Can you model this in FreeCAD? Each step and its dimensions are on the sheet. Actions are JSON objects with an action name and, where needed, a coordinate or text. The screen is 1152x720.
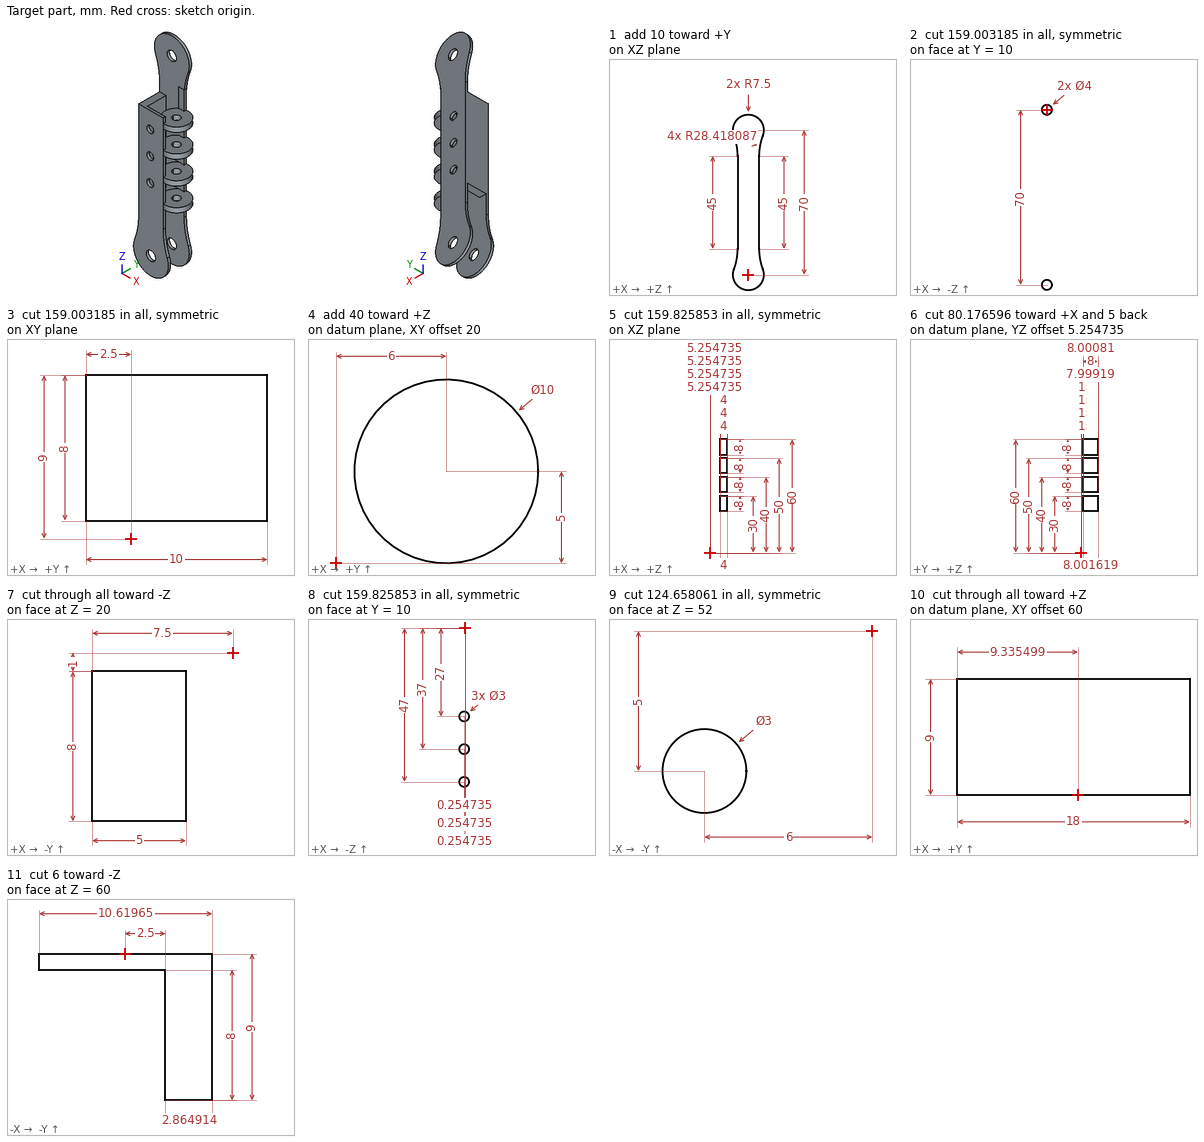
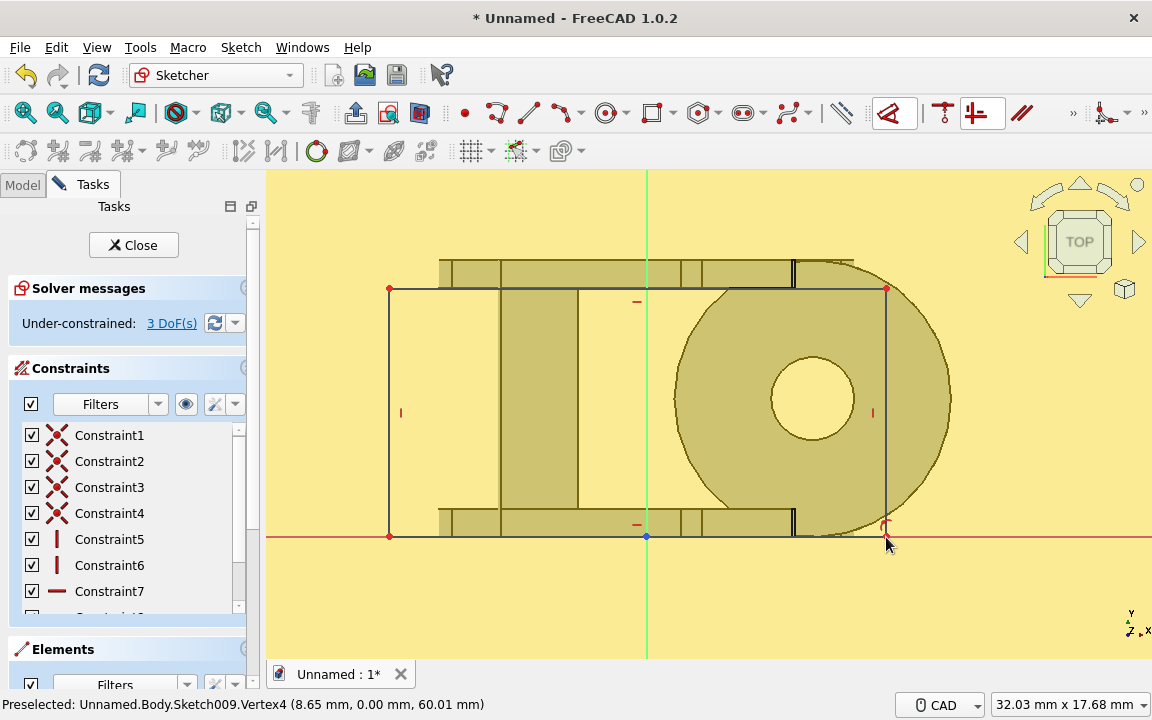
{"action": "left_click", "coordinate": [389, 363]}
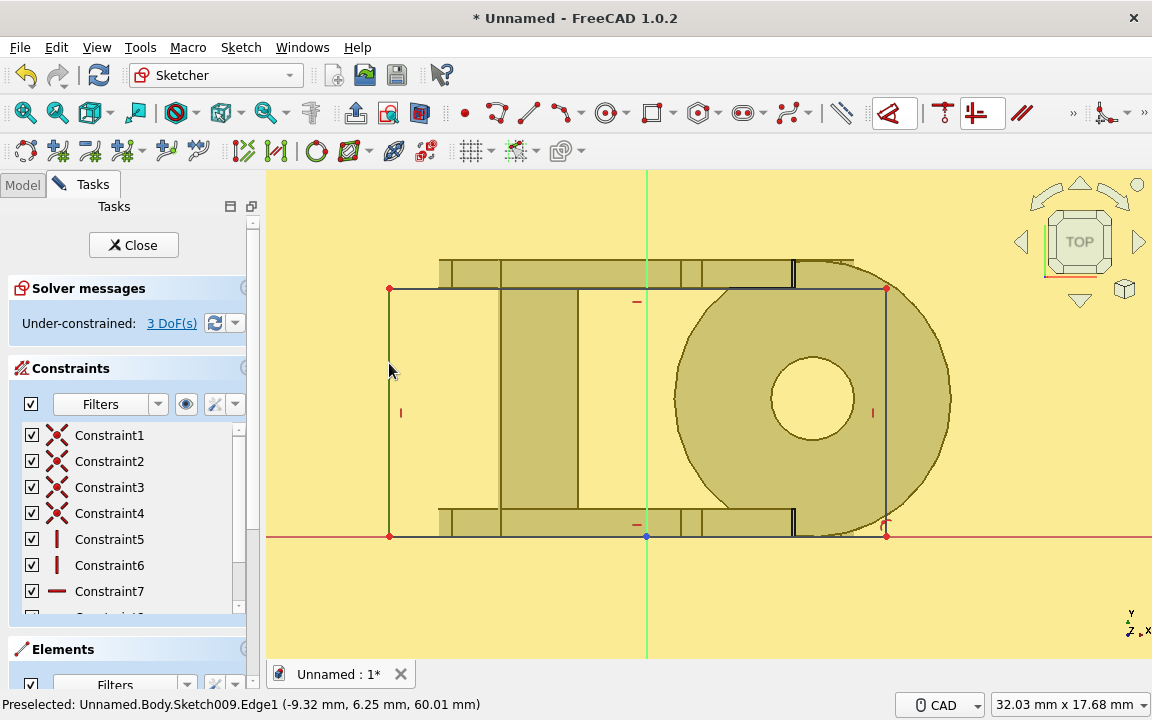
{"action": "key", "text": "i"}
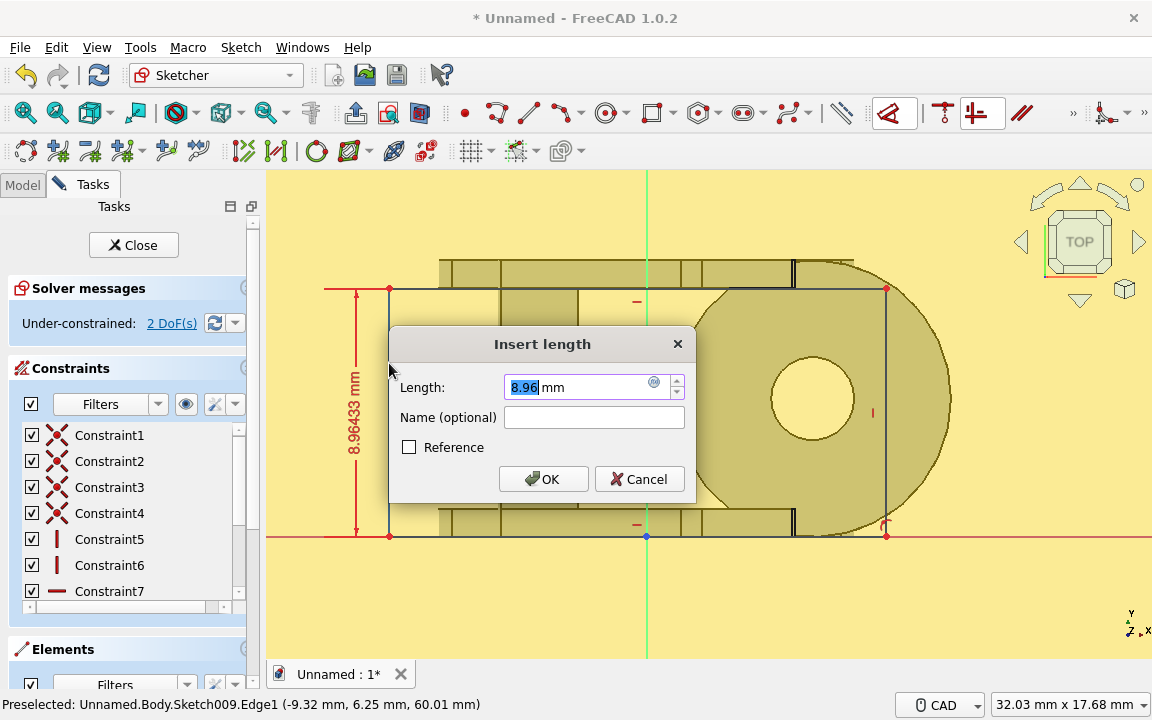
{"action": "type", "text": "9"}
{"action": "key", "text": "Return"}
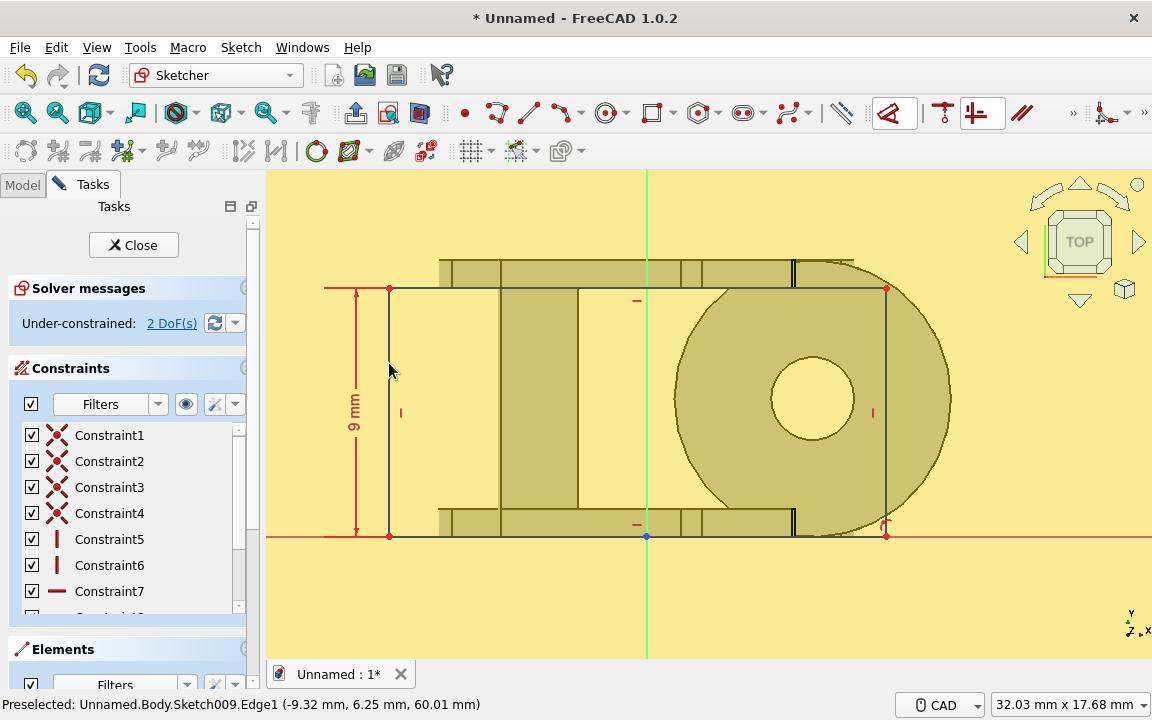
{"action": "left_click", "coordinate": [538, 537]}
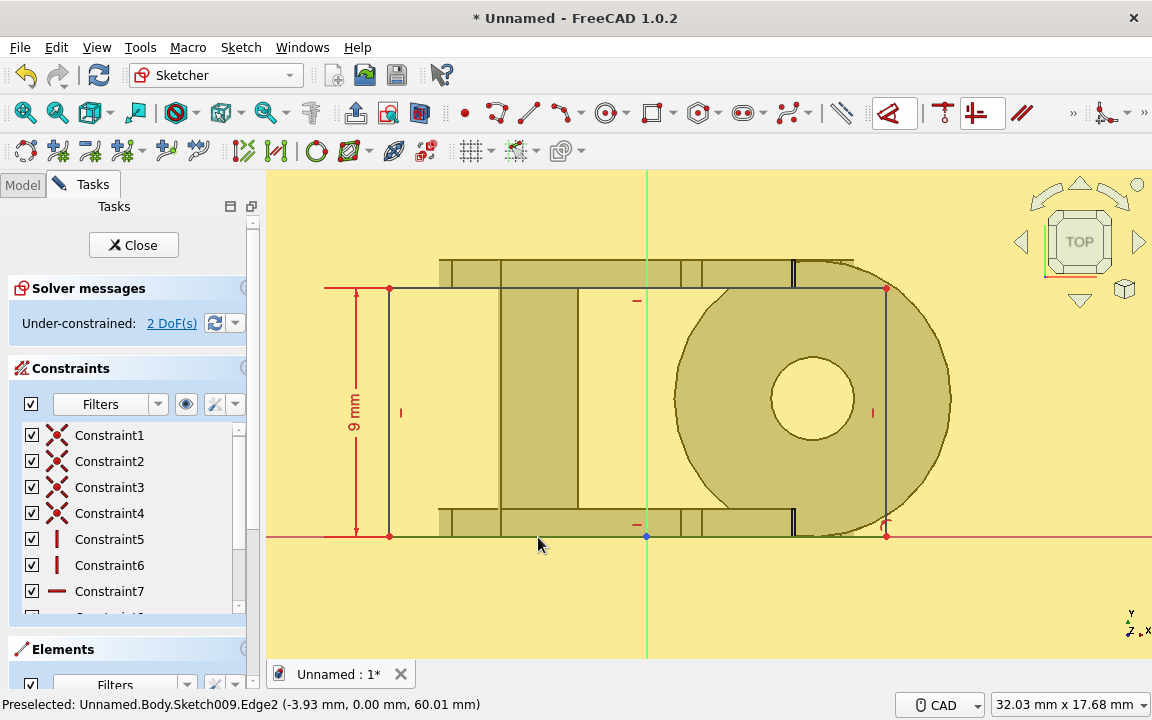
{"action": "key", "text": "l"}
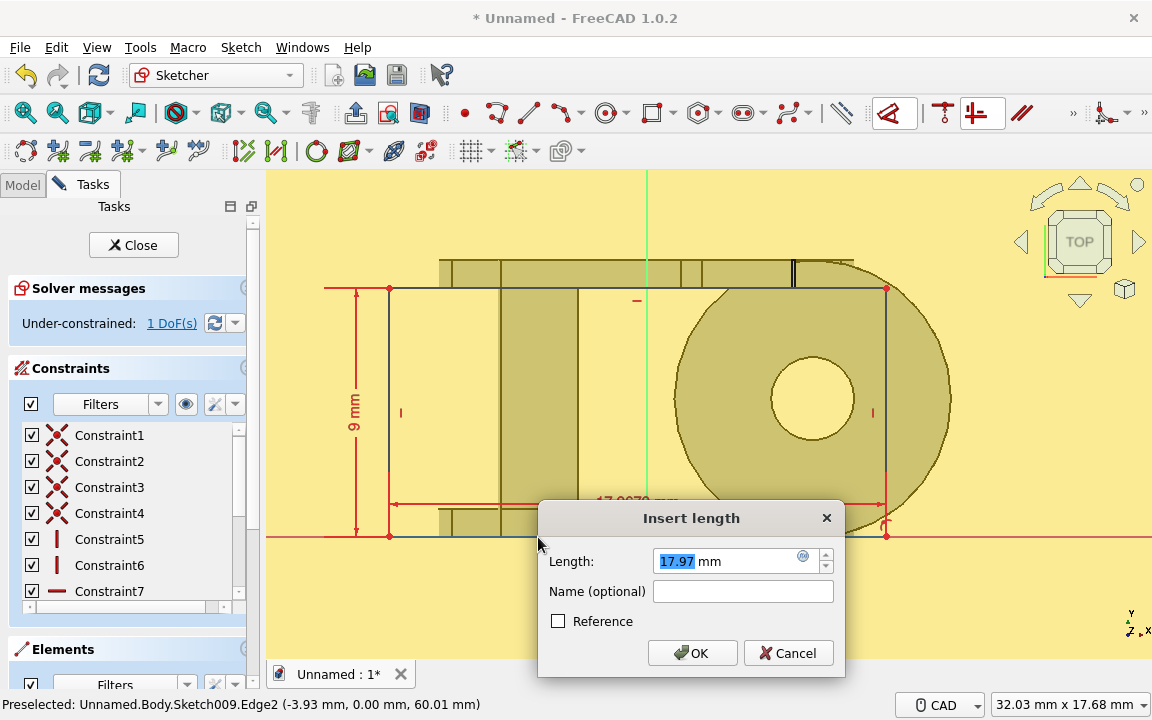
{"action": "type", "text": "18"}
{"action": "key", "text": "Return"}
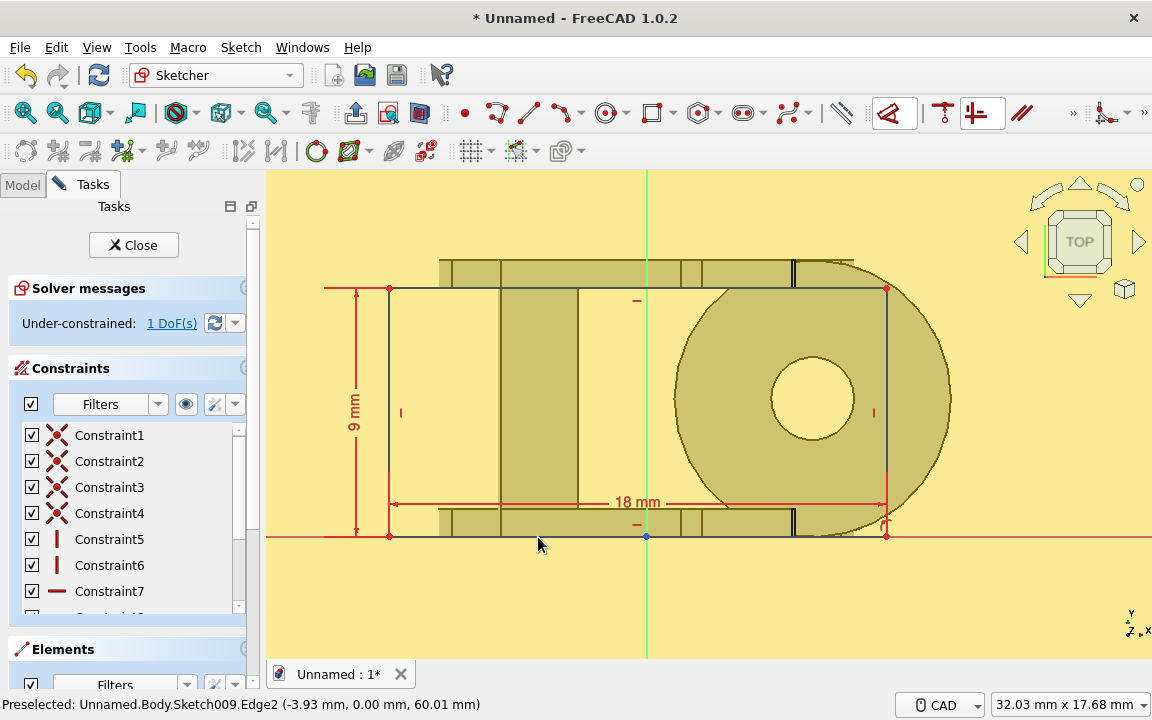
{"action": "left_click", "coordinate": [389, 288]}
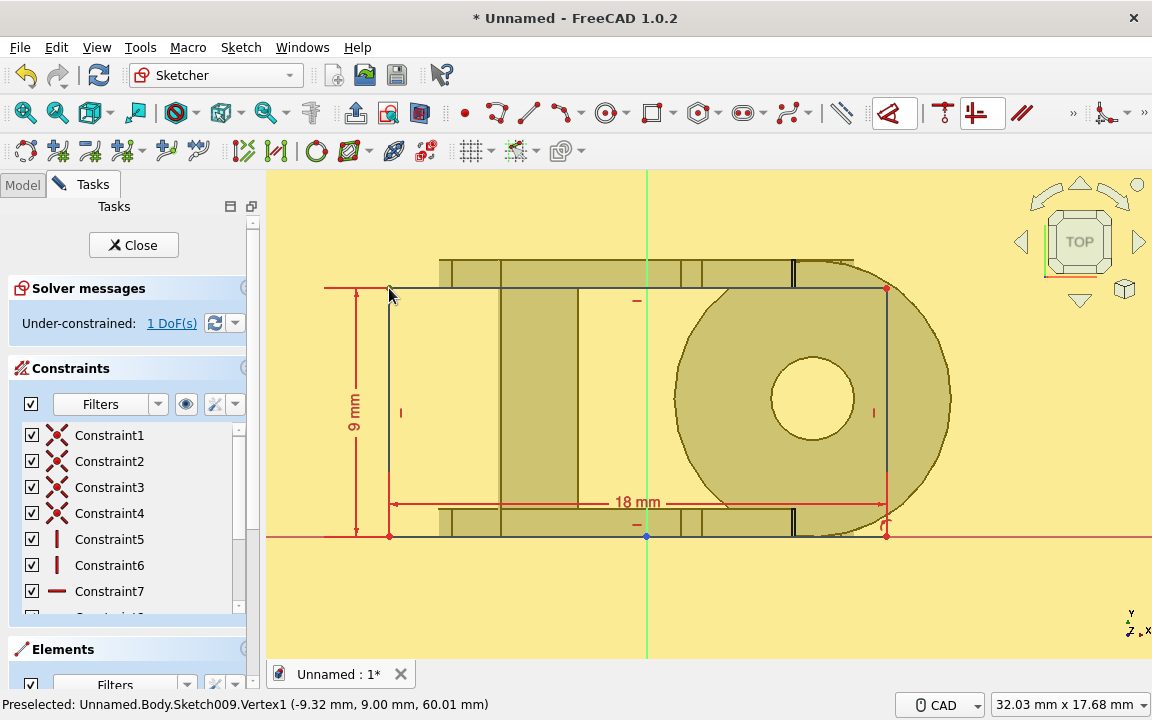
{"action": "key", "text": "l"}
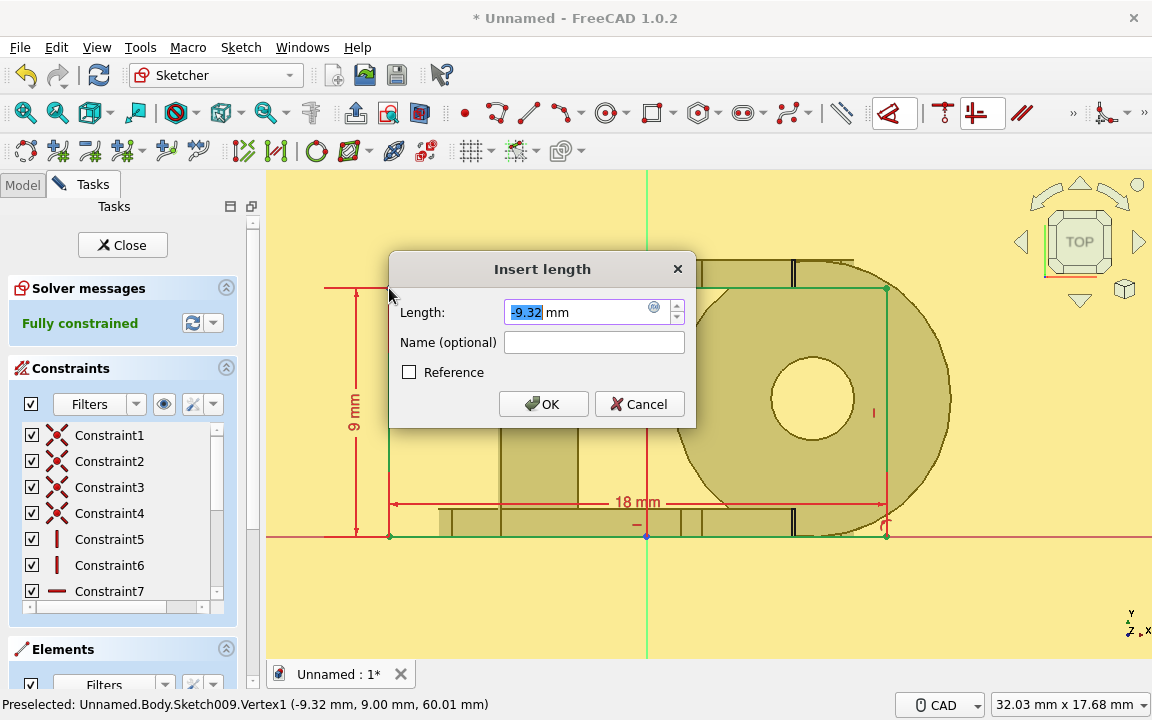
{"action": "type", "text": "-9.335499"}
{"action": "key", "text": "Return"}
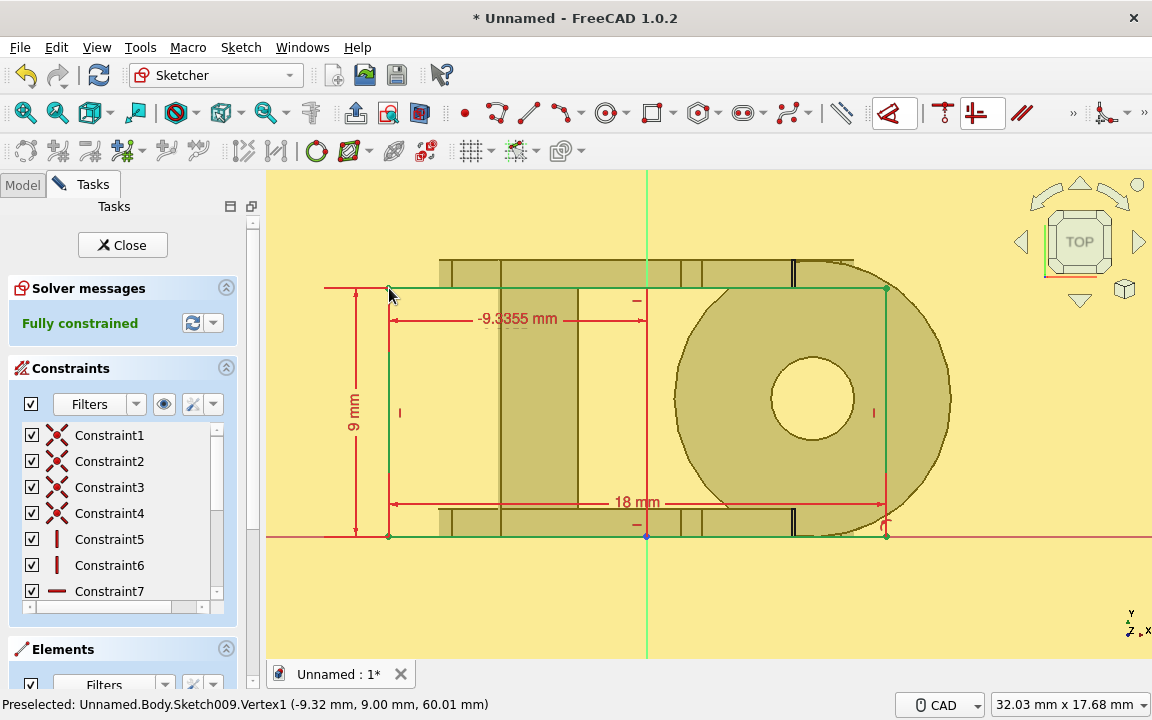
{"action": "left_click", "coordinate": [123, 245]}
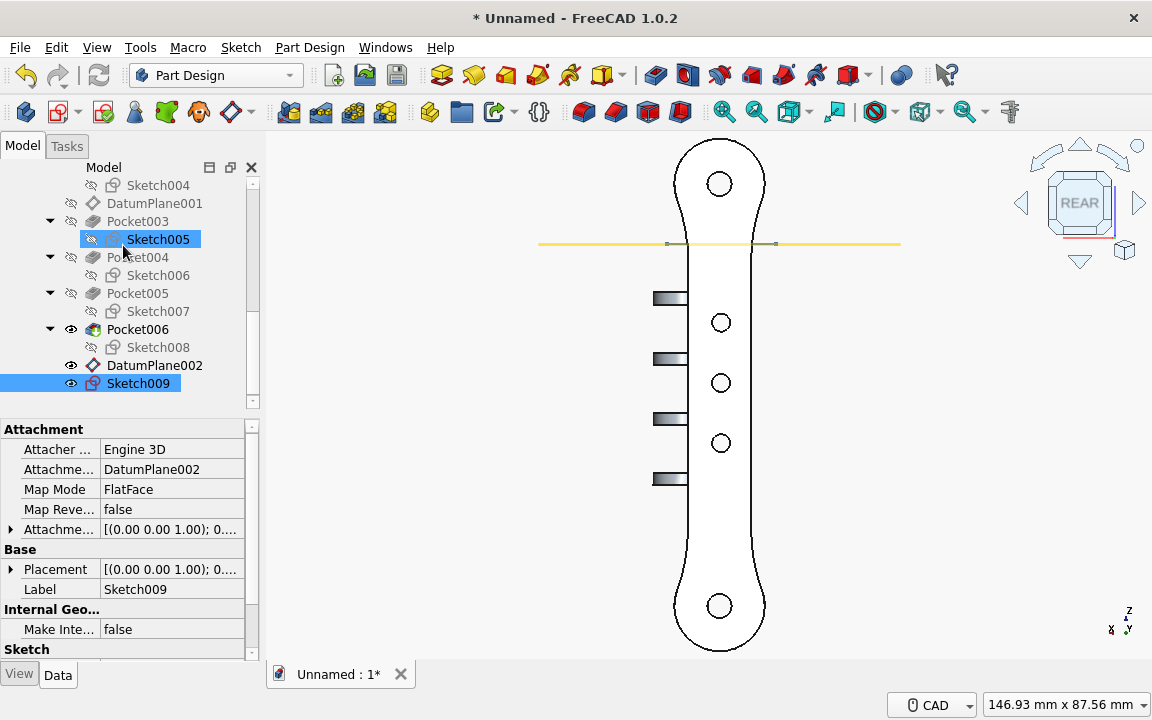
{"action": "left_click", "coordinate": [656, 76]}